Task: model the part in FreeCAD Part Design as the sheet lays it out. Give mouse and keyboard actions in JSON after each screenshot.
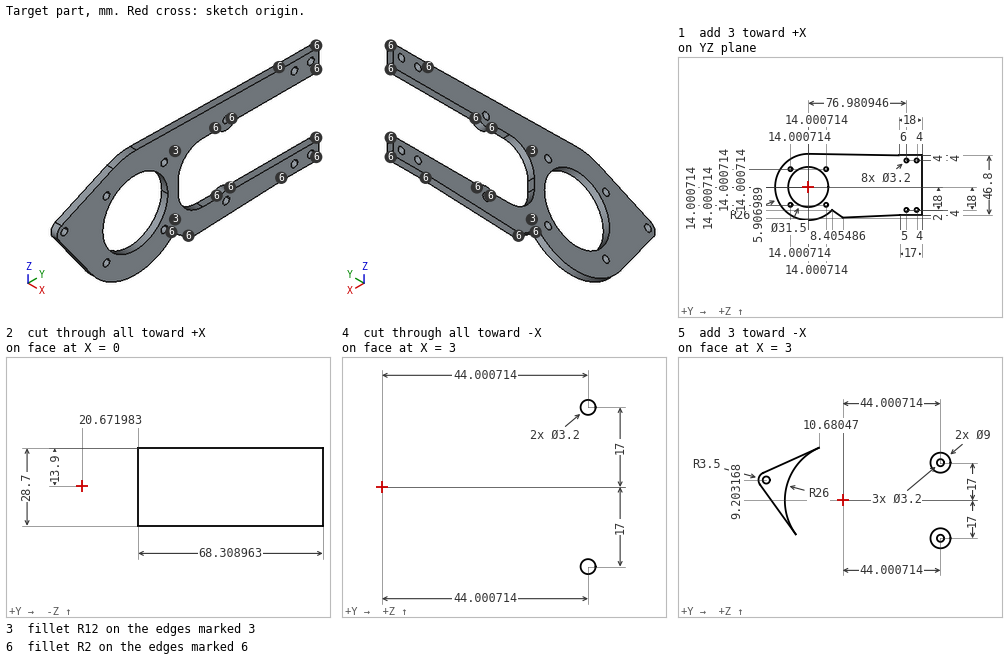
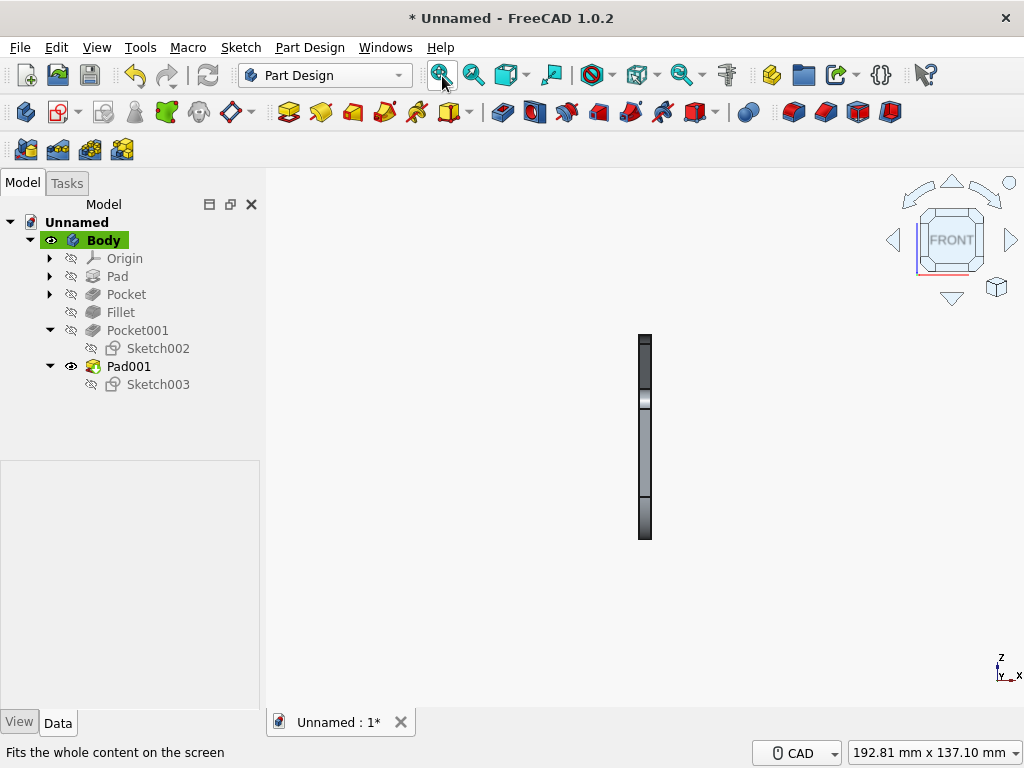
{"action": "left_click", "coordinate": [442, 76]}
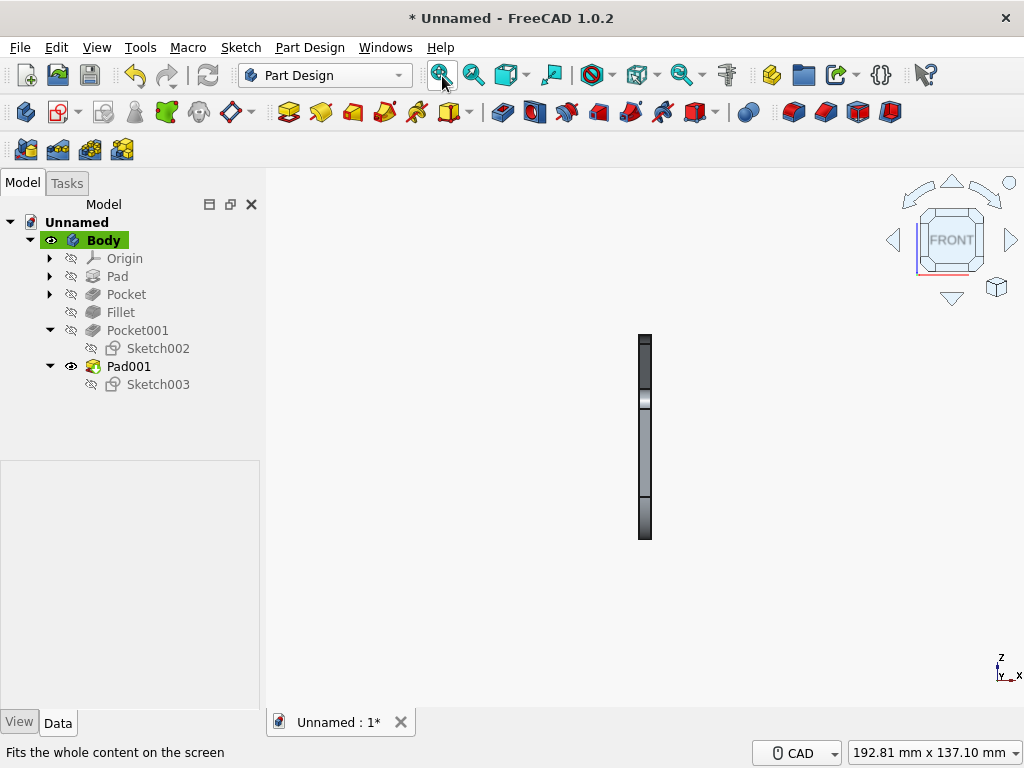
{"action": "scroll", "coordinate": [645, 378], "scroll_direction": "up", "scroll_amount": 7}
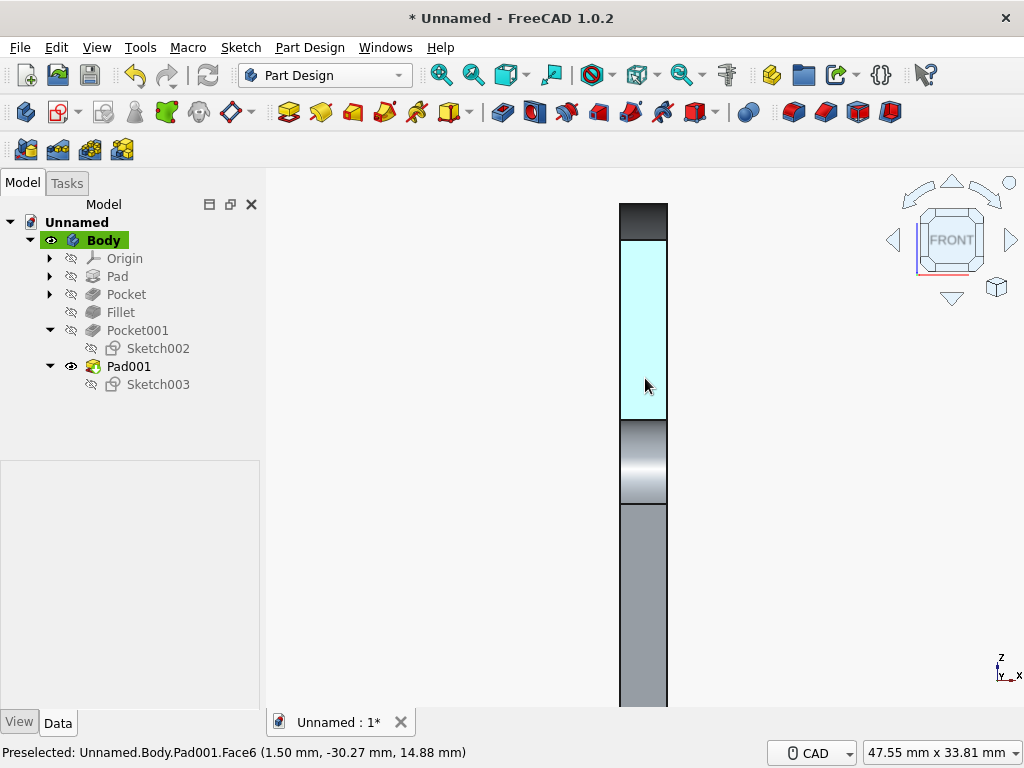
{"action": "left_click", "coordinate": [442, 76]}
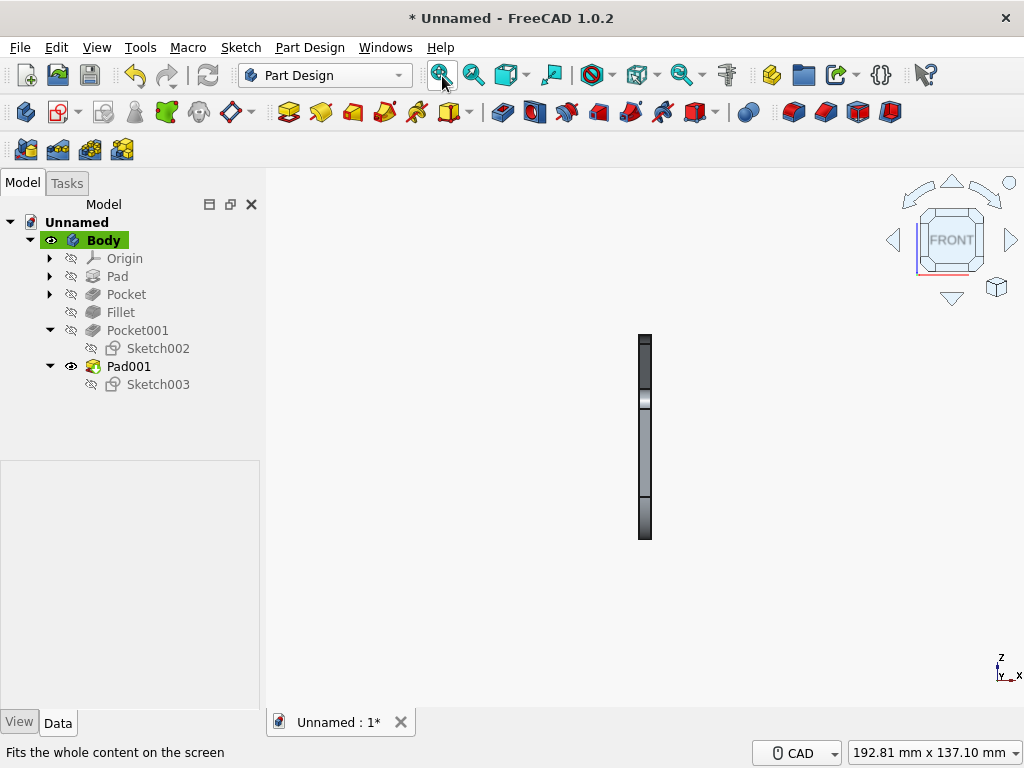
{"action": "key", "text": "3"}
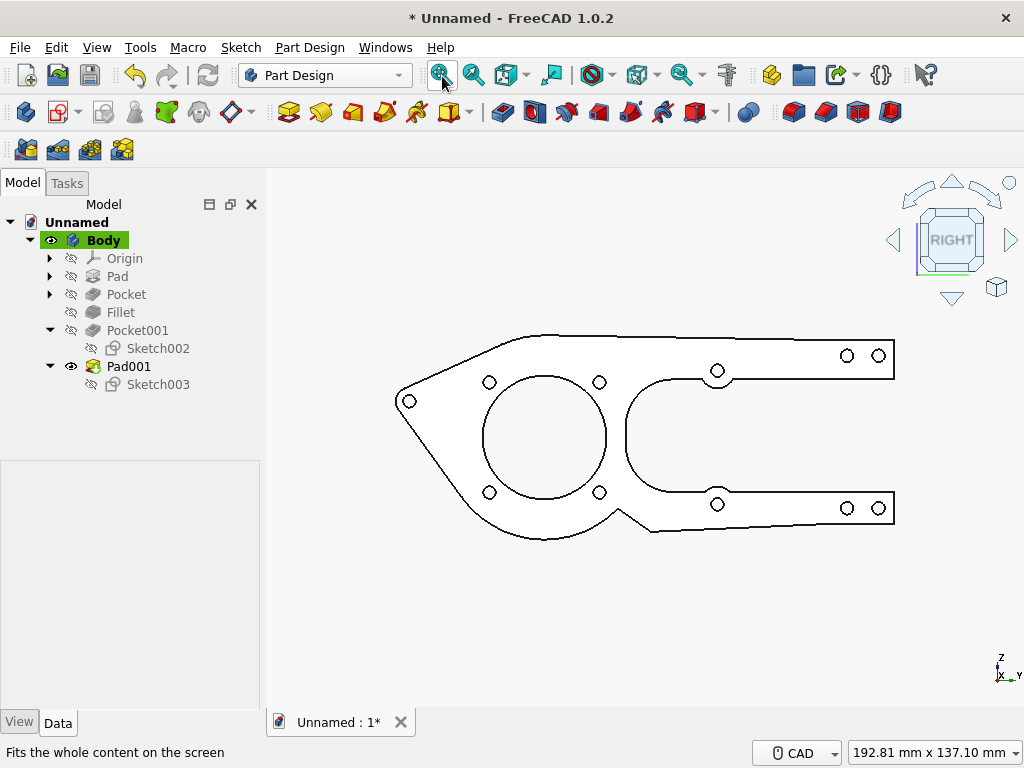
{"action": "scroll", "coordinate": [733, 378], "scroll_direction": "up", "scroll_amount": 7}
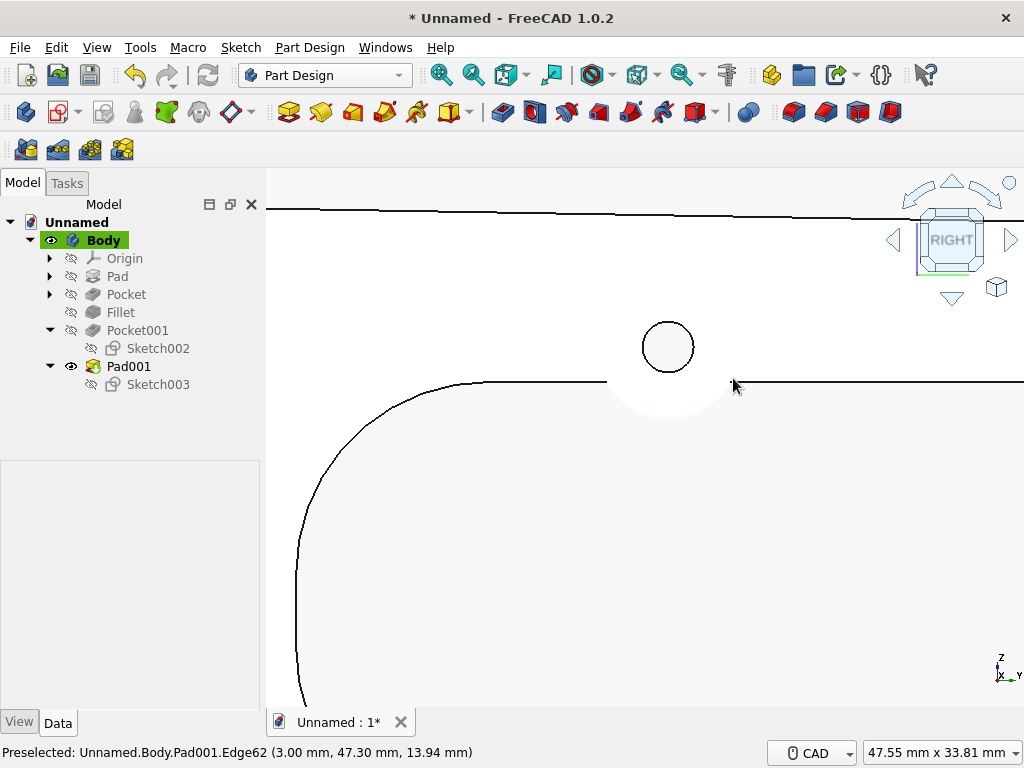
{"action": "left_click", "coordinate": [442, 76]}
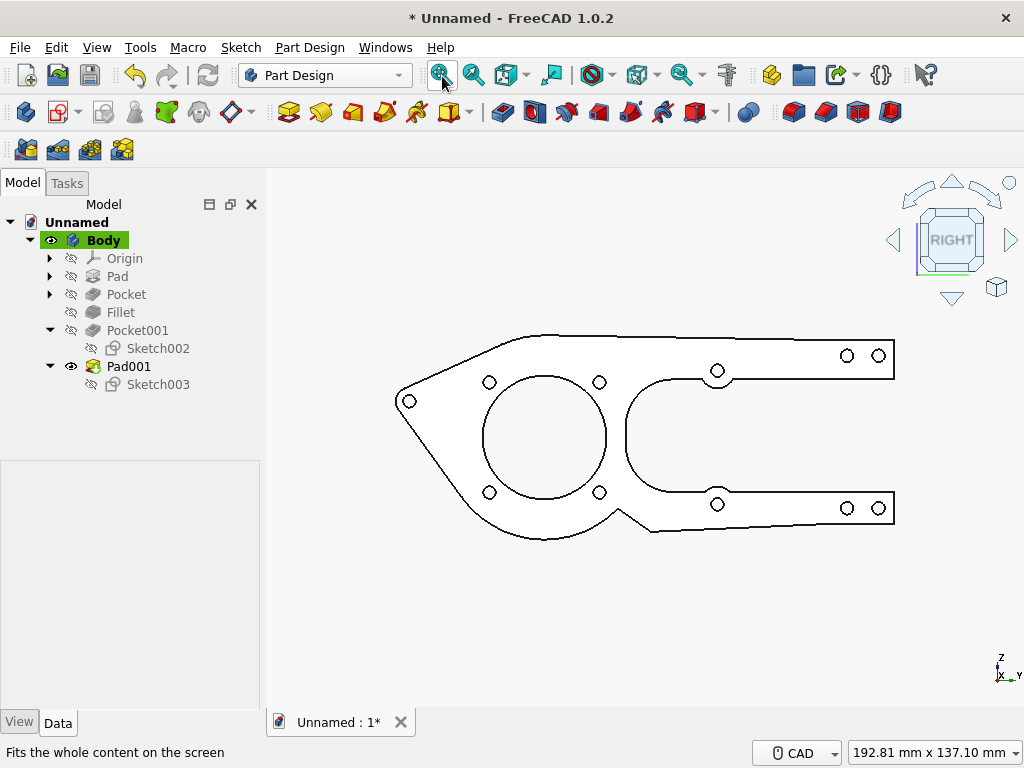
{"action": "key", "text": "5"}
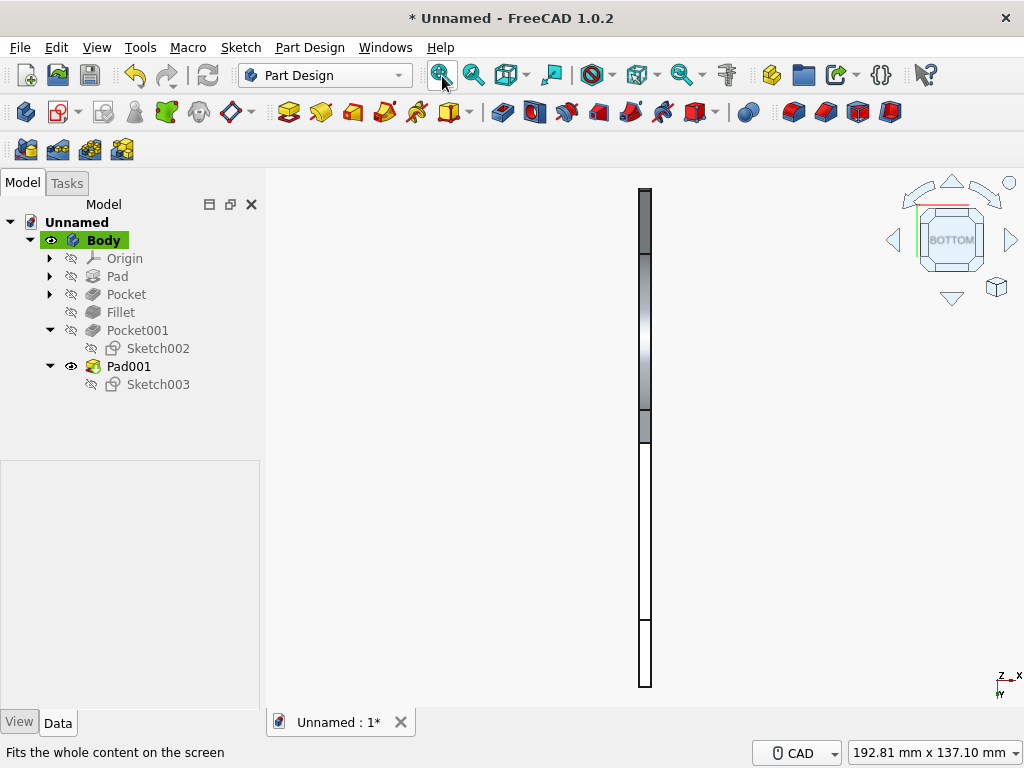
{"action": "scroll", "coordinate": [645, 524], "scroll_direction": "up", "scroll_amount": 7}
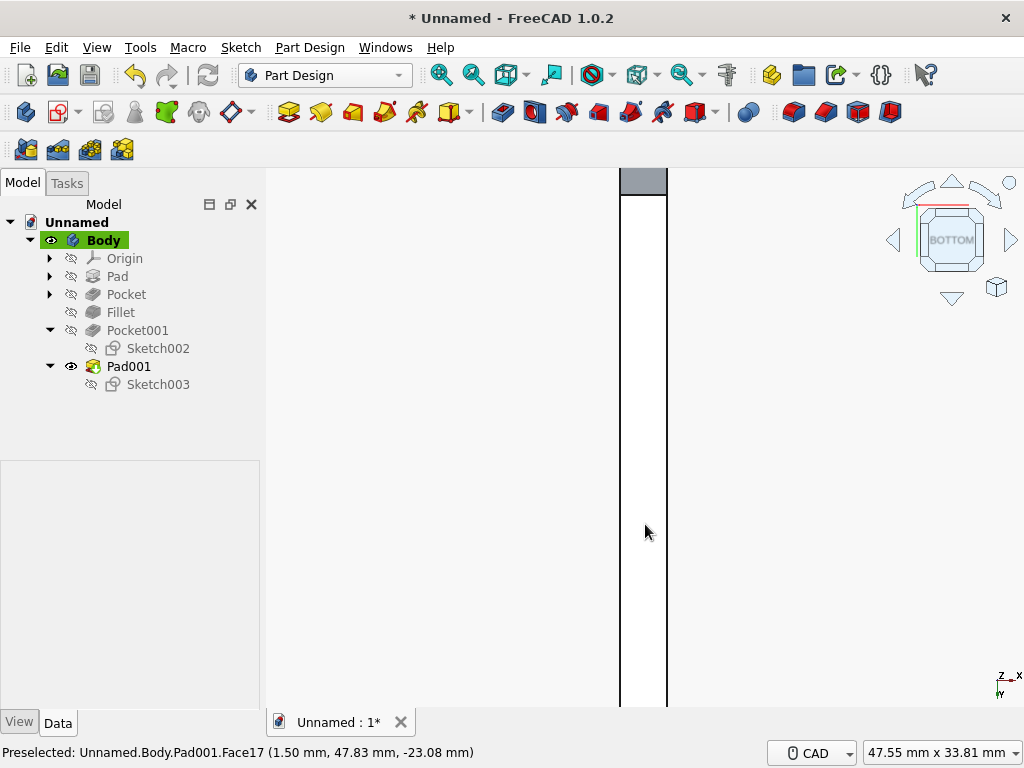
{"action": "left_click", "coordinate": [442, 76]}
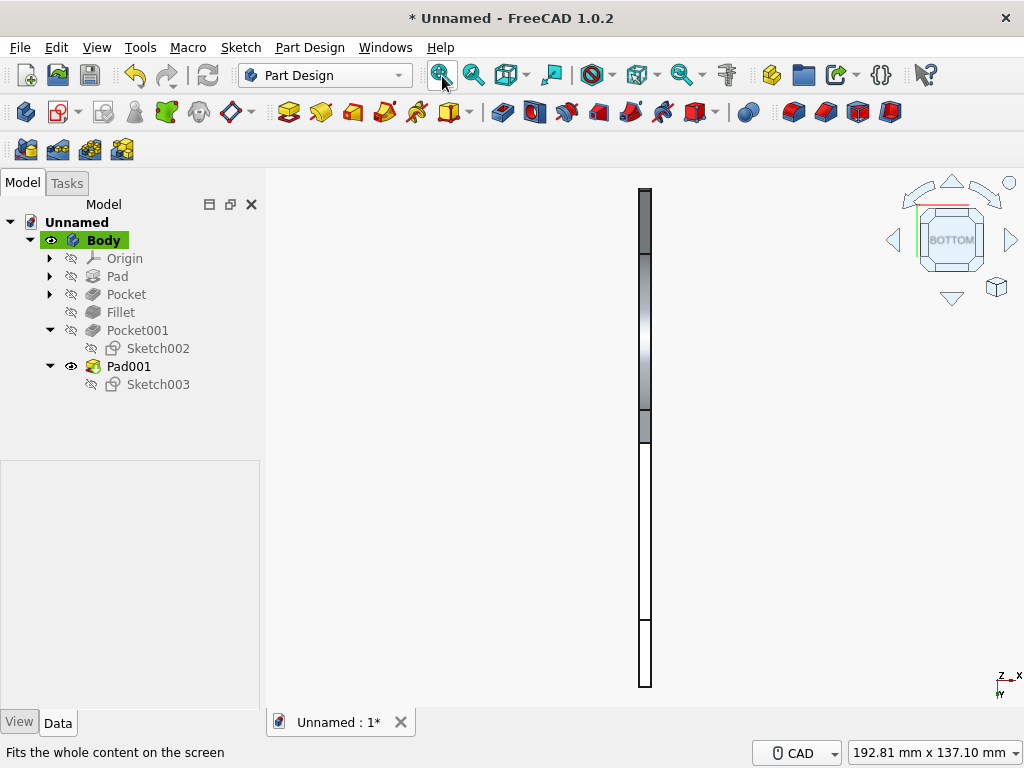
{"action": "key", "text": "4"}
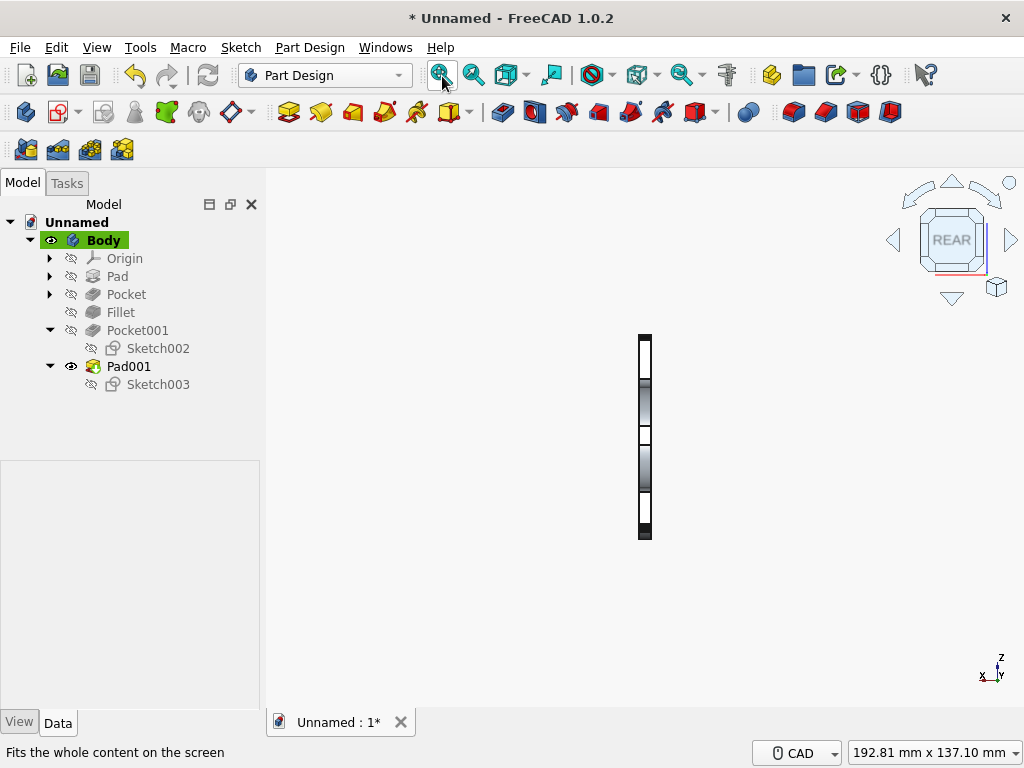
{"action": "left_click", "coordinate": [442, 76]}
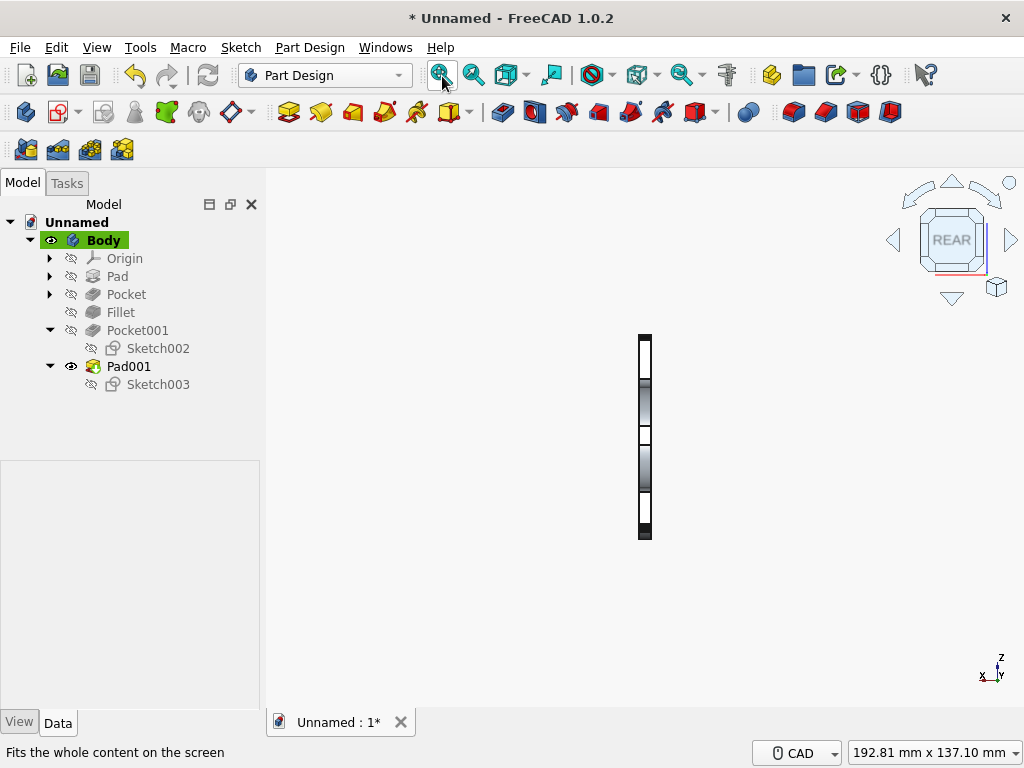
{"action": "scroll", "coordinate": [645, 378], "scroll_direction": "up", "scroll_amount": 7}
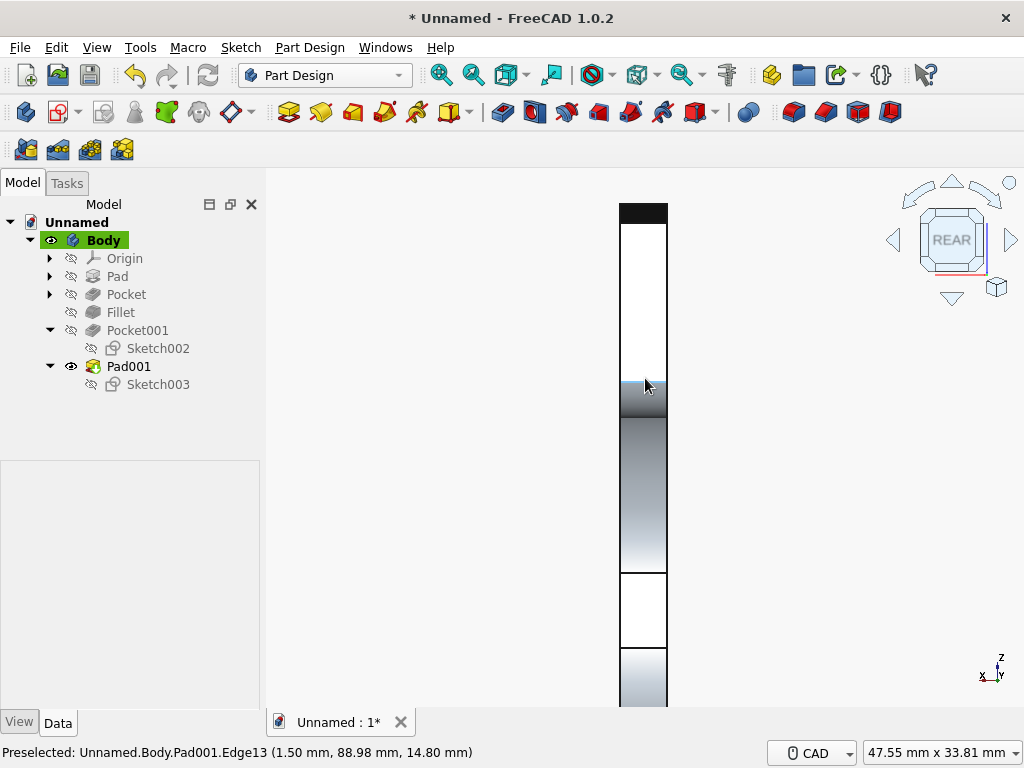
{"action": "left_click", "coordinate": [643, 222]}